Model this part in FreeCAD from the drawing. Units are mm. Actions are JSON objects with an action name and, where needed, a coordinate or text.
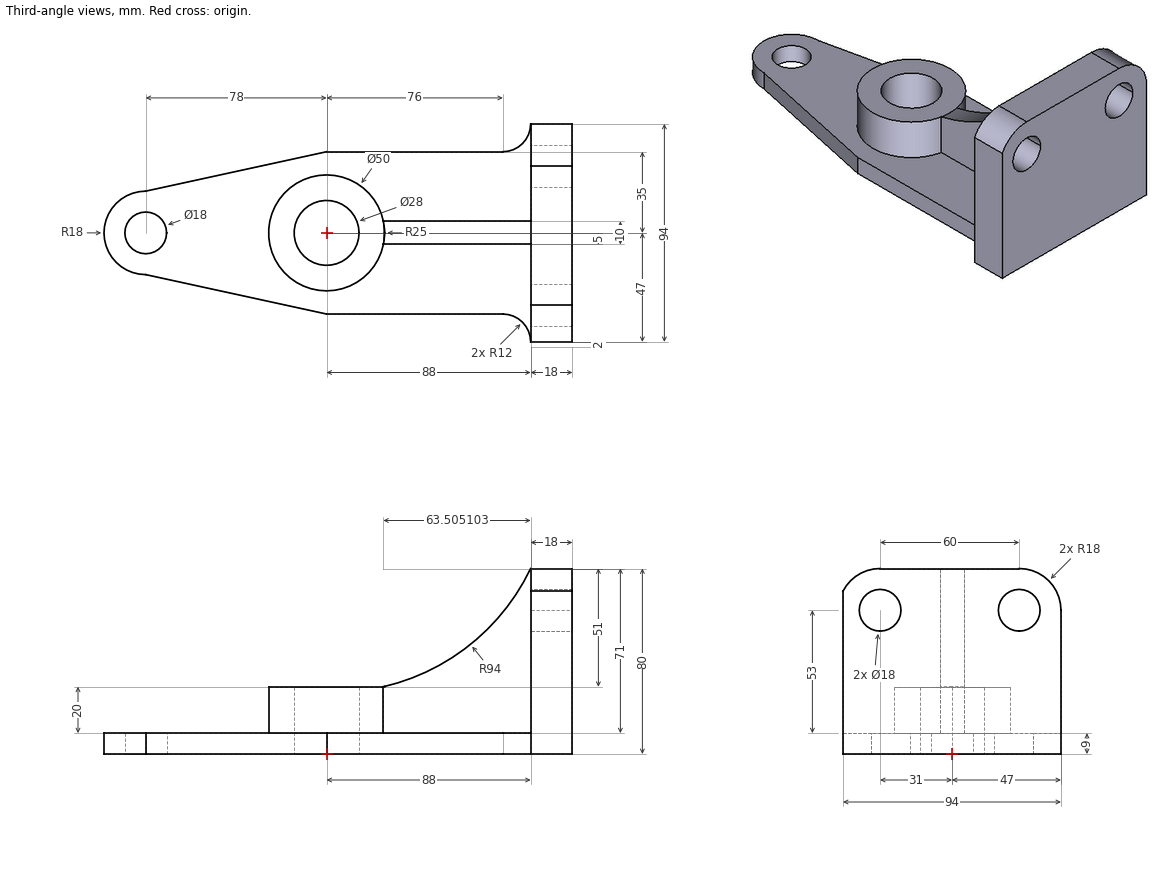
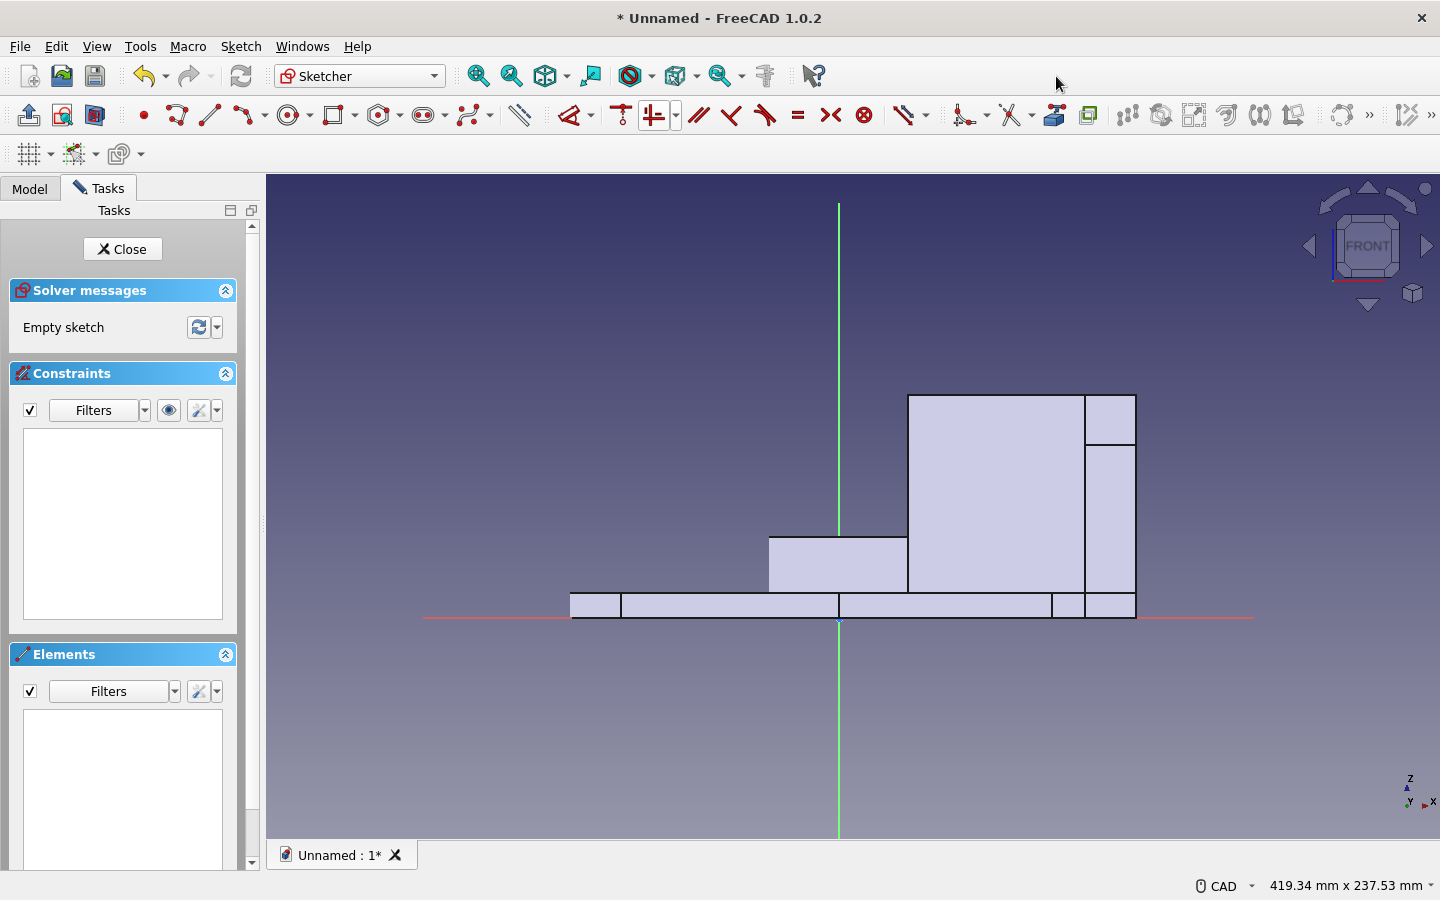
{"action": "scroll", "coordinate": [1178, 507], "scroll_direction": "up", "scroll_amount": 3}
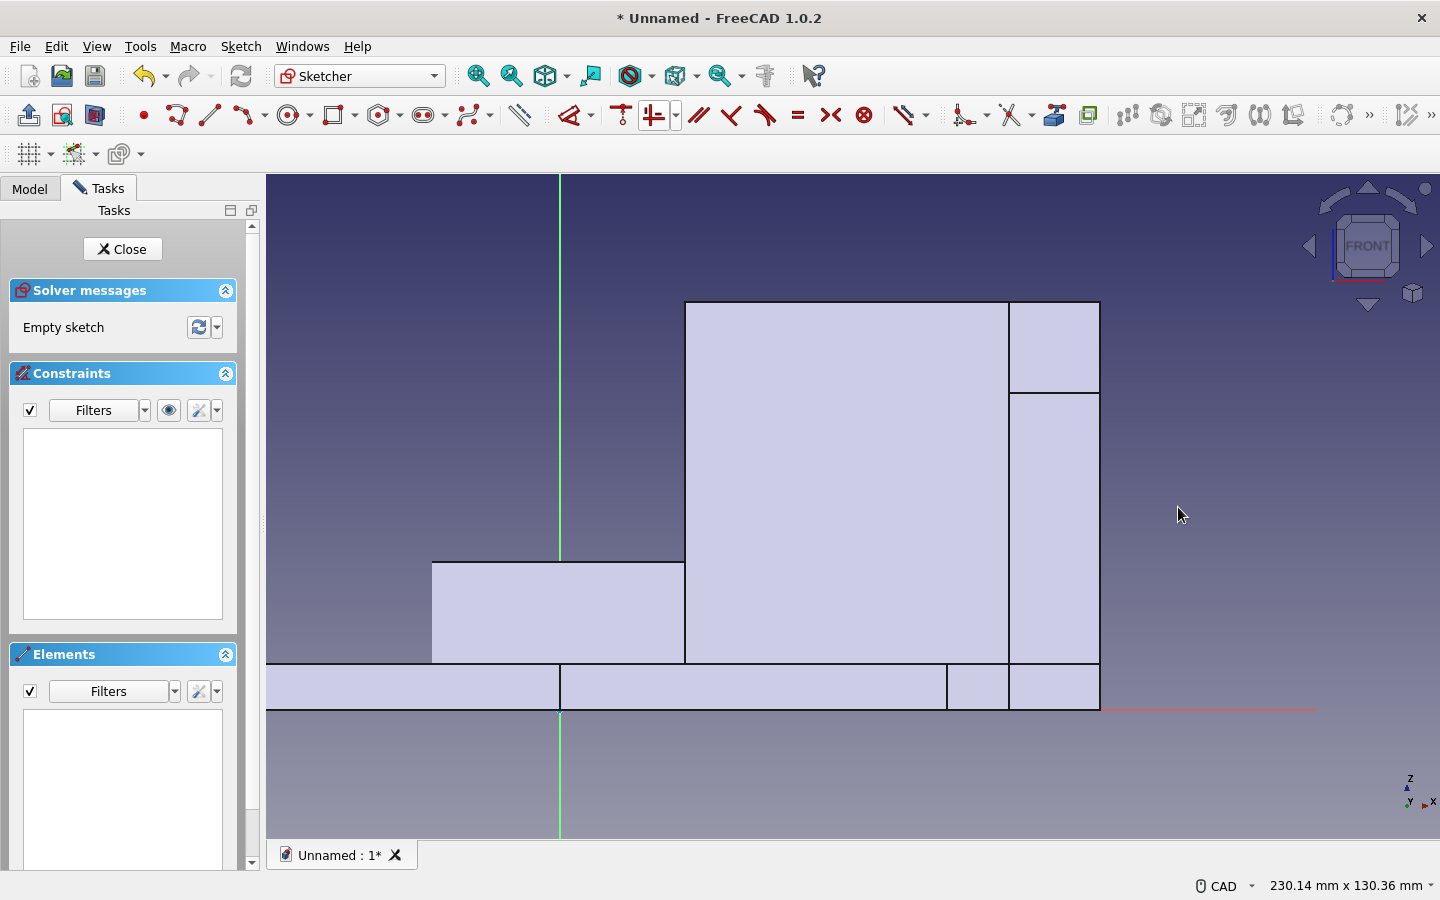
{"action": "left_click", "coordinate": [177, 116]}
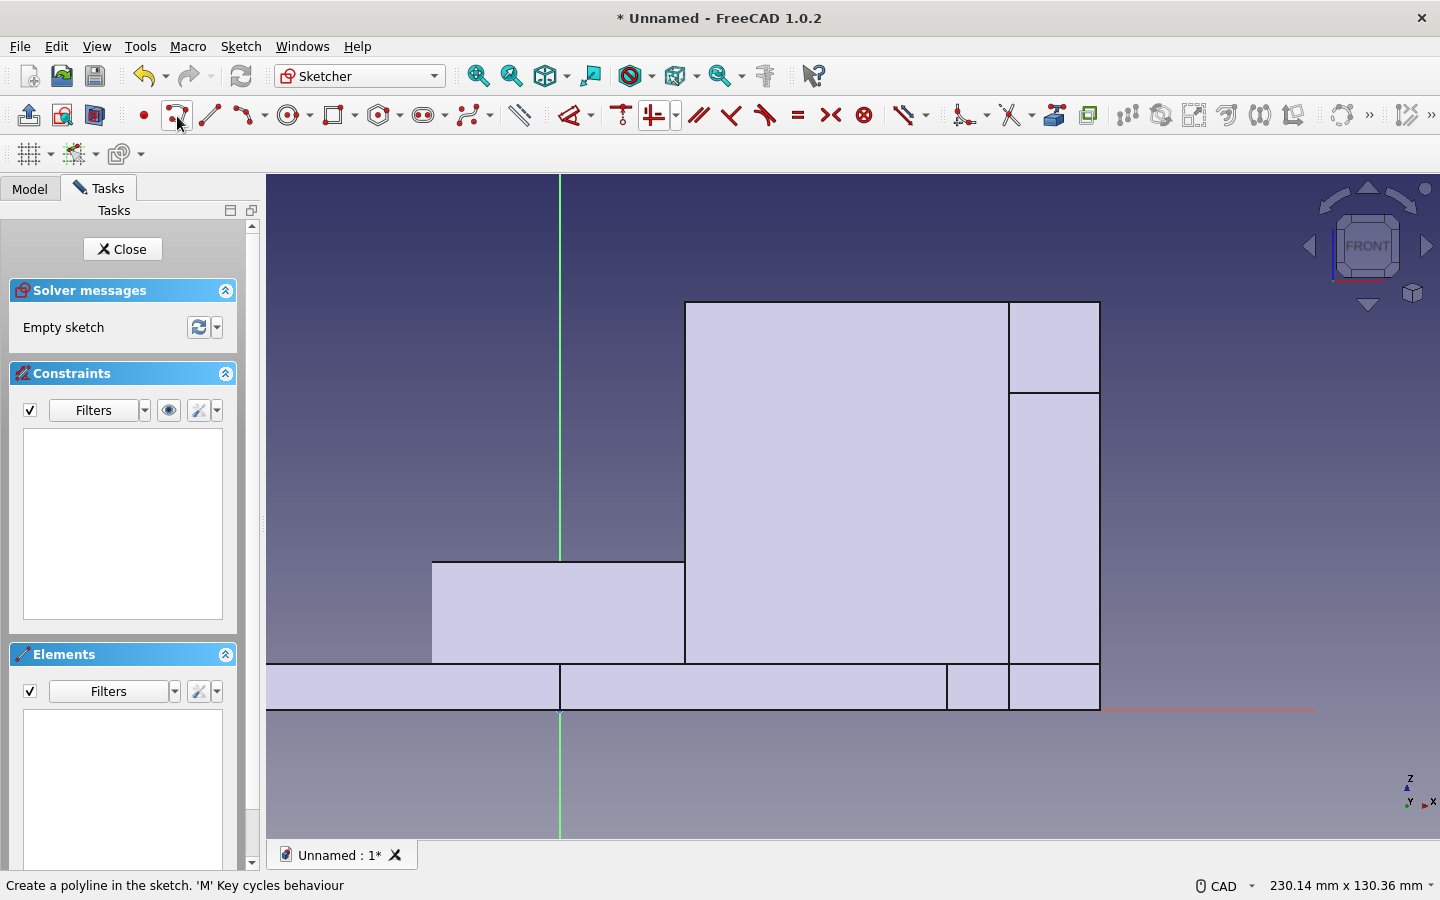
{"action": "left_click", "coordinate": [1009, 302]}
{"action": "left_click", "coordinate": [685, 302]}
{"action": "left_click", "coordinate": [685, 562]}
{"action": "right_click", "coordinate": [685, 562]}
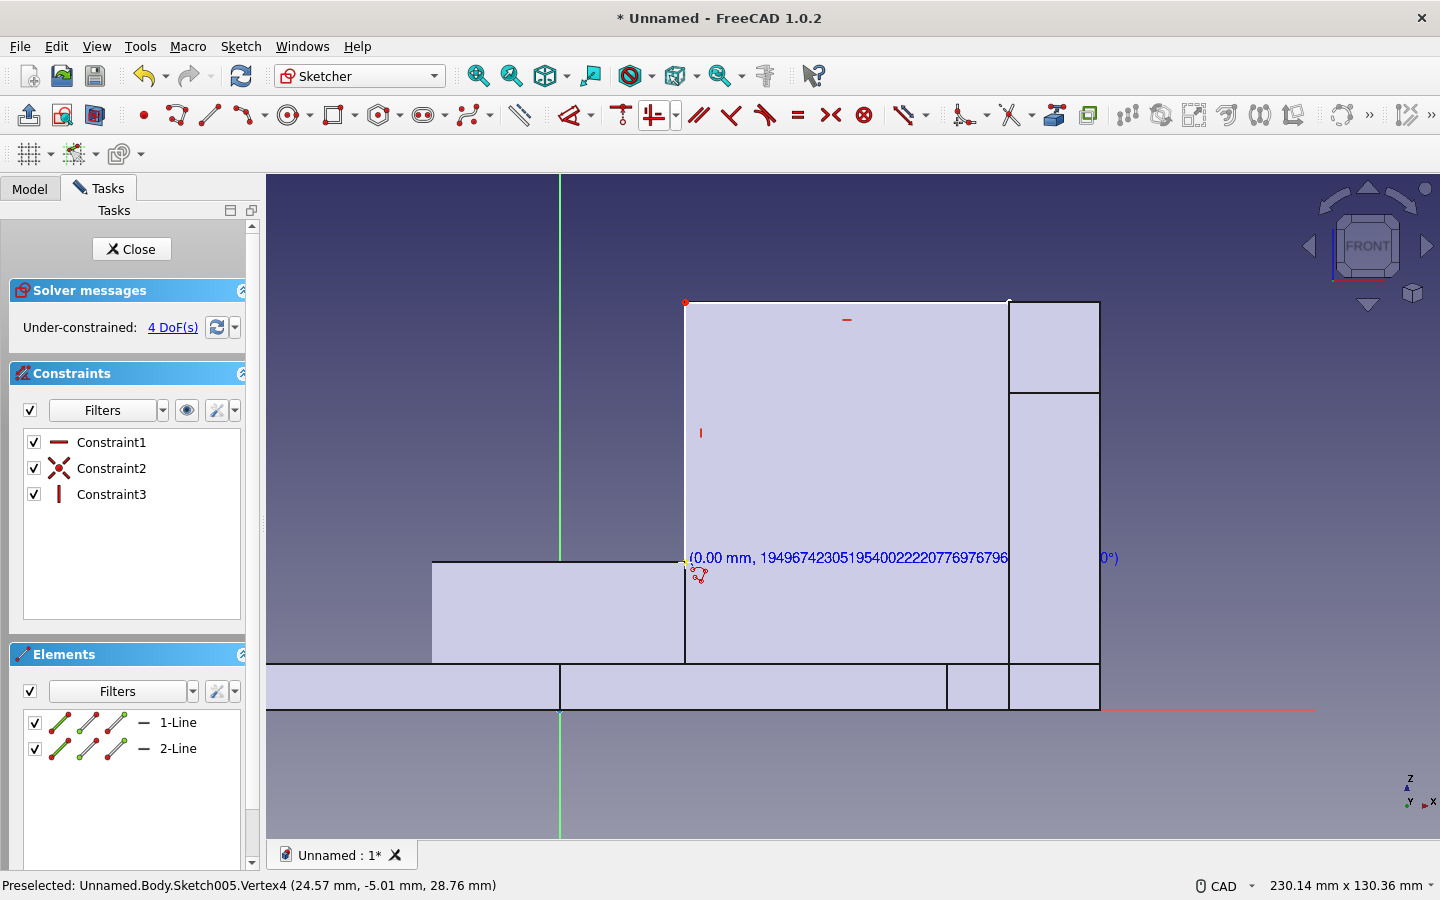
{"action": "left_click", "coordinate": [242, 116]}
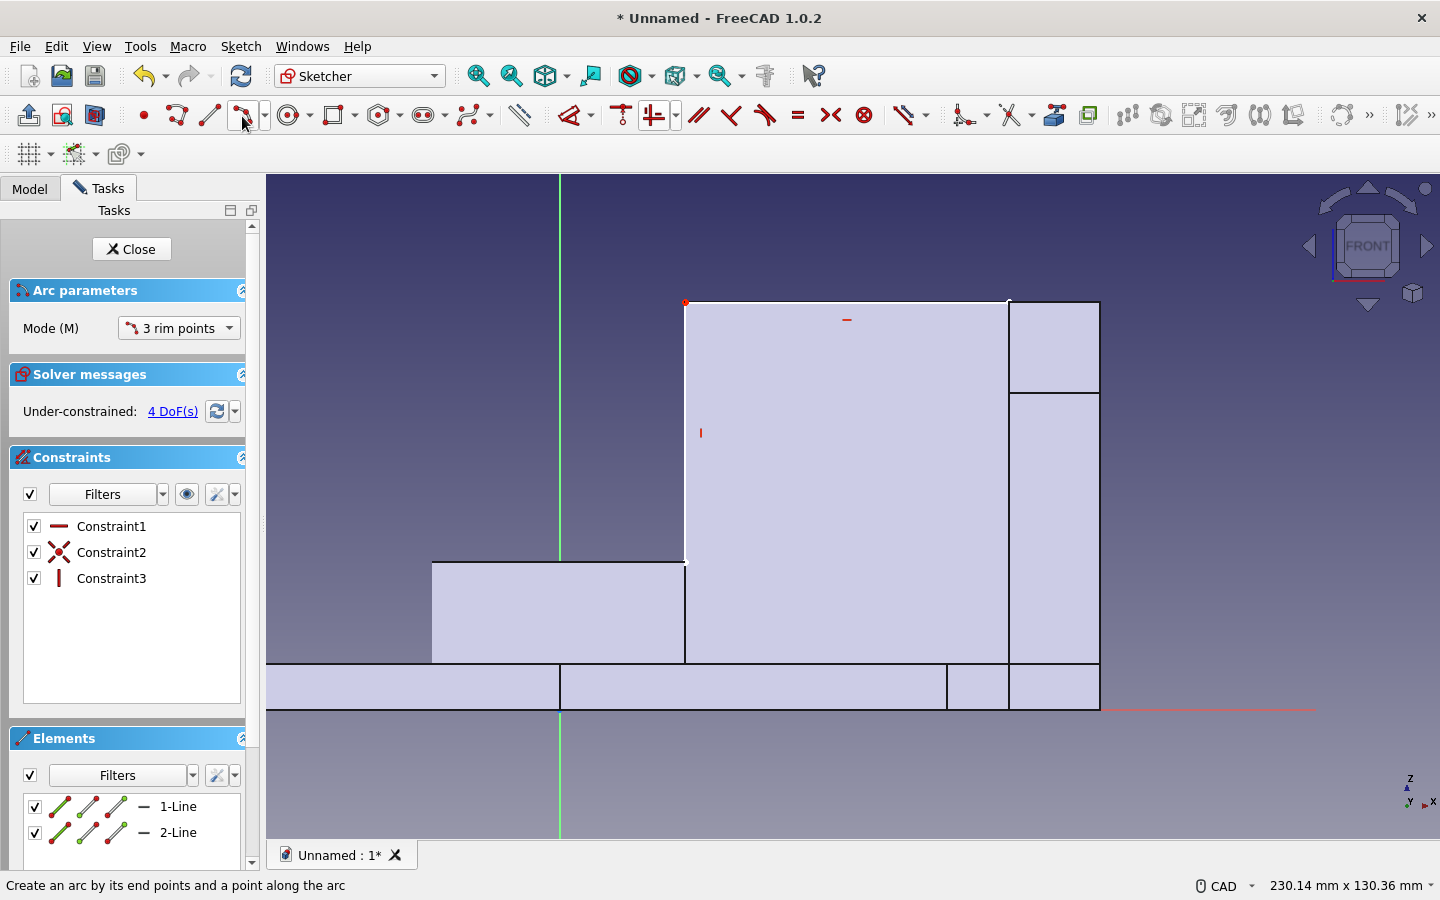
{"action": "left_click", "coordinate": [685, 563]}
{"action": "left_click", "coordinate": [1009, 303]}
{"action": "left_click", "coordinate": [876, 469]}
{"action": "key", "text": "Escape"}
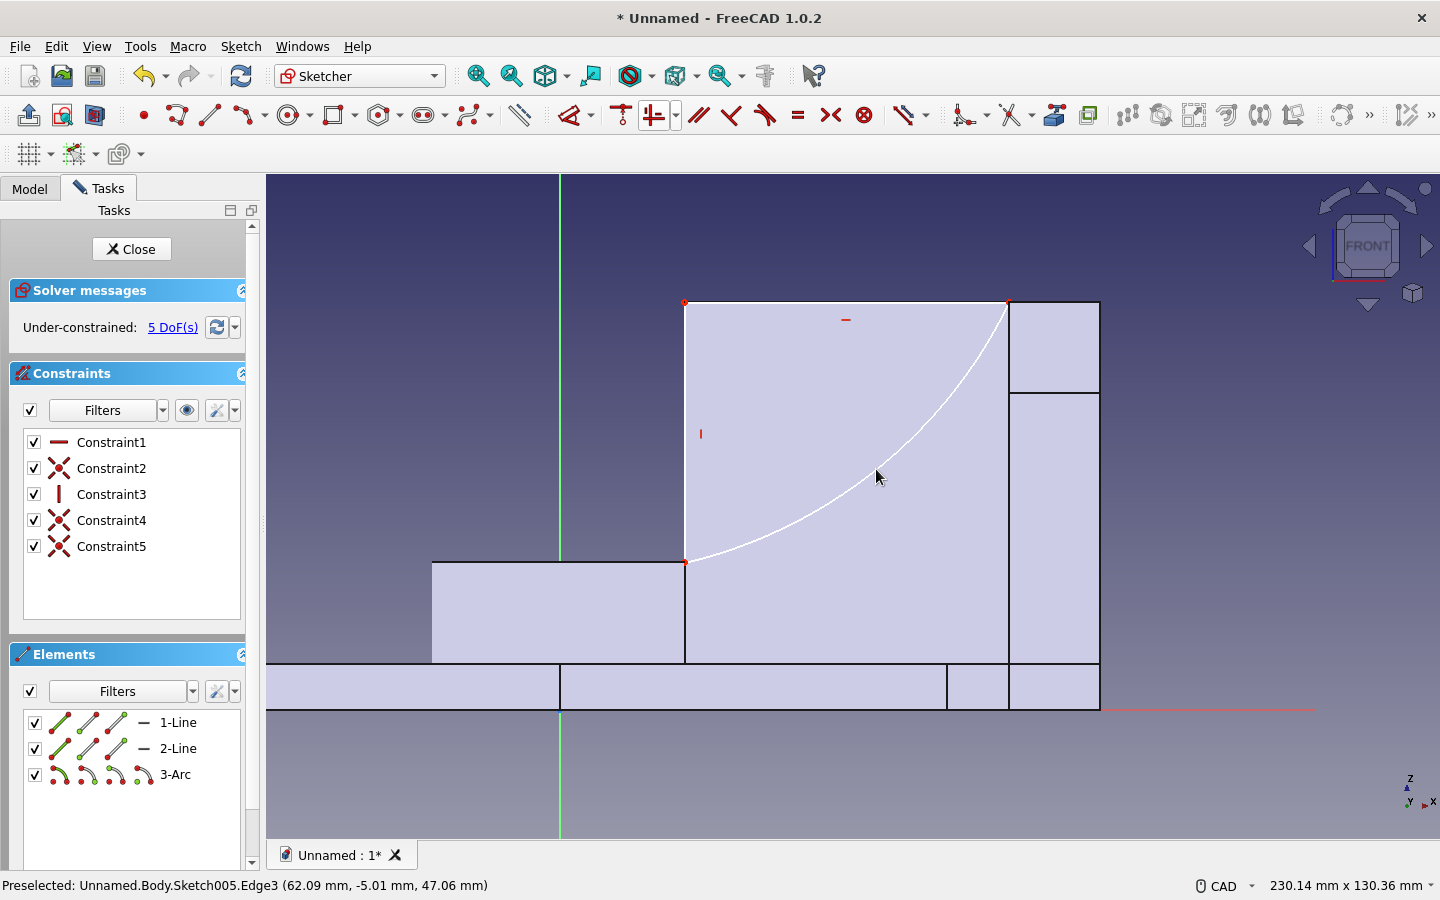
{"action": "left_click", "coordinate": [568, 116]}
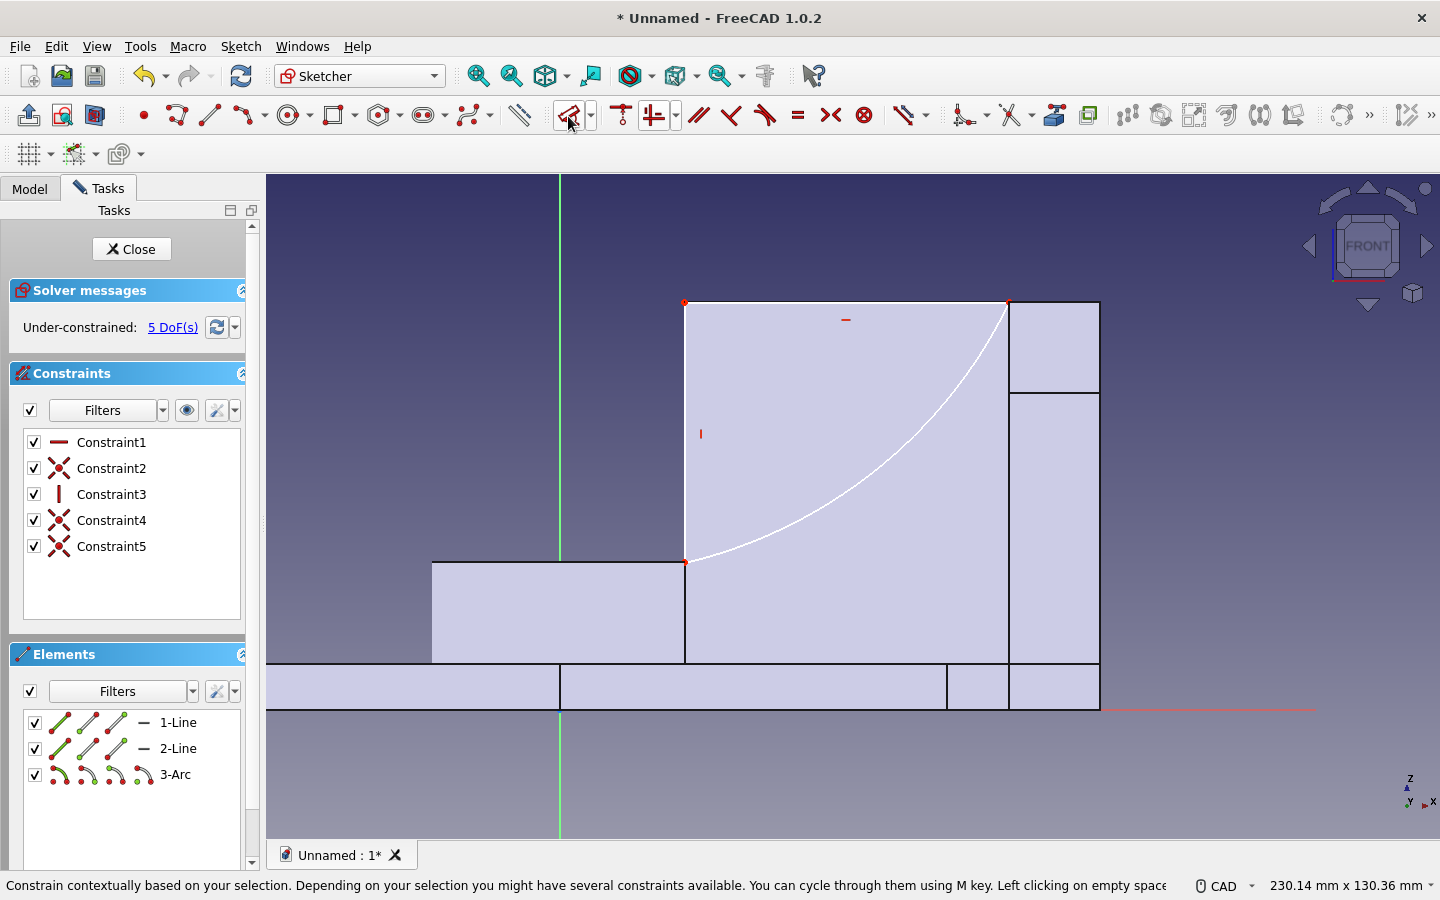
{"action": "left_click", "coordinate": [805, 517]}
{"action": "left_click", "coordinate": [820, 545]}